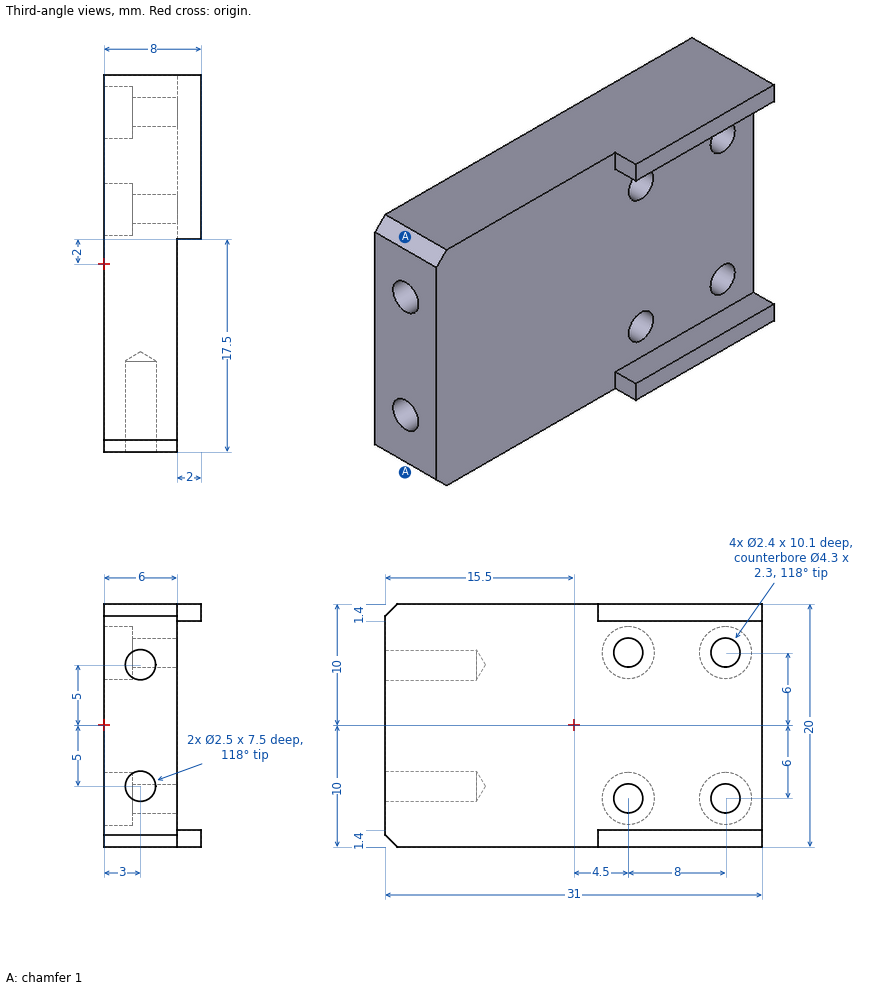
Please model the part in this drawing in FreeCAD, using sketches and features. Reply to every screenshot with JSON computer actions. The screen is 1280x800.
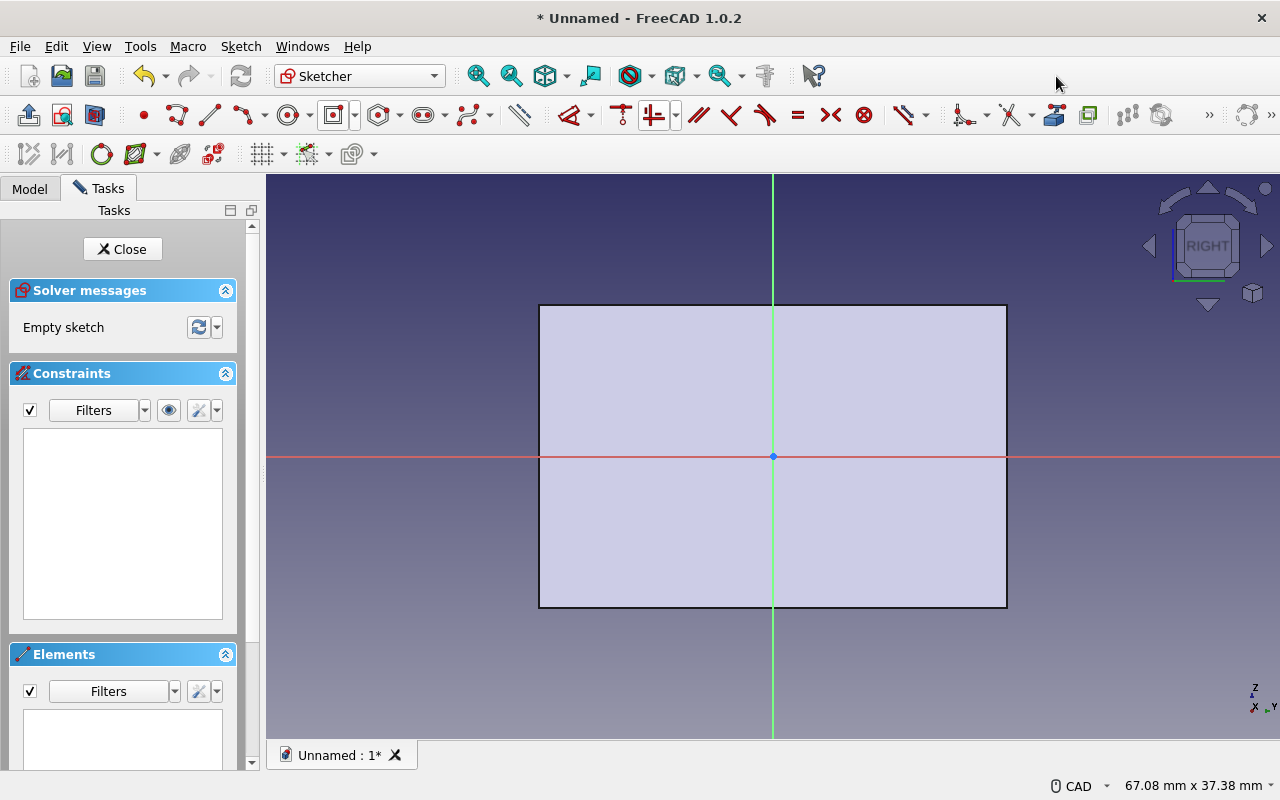
{"action": "key", "text": "g r"}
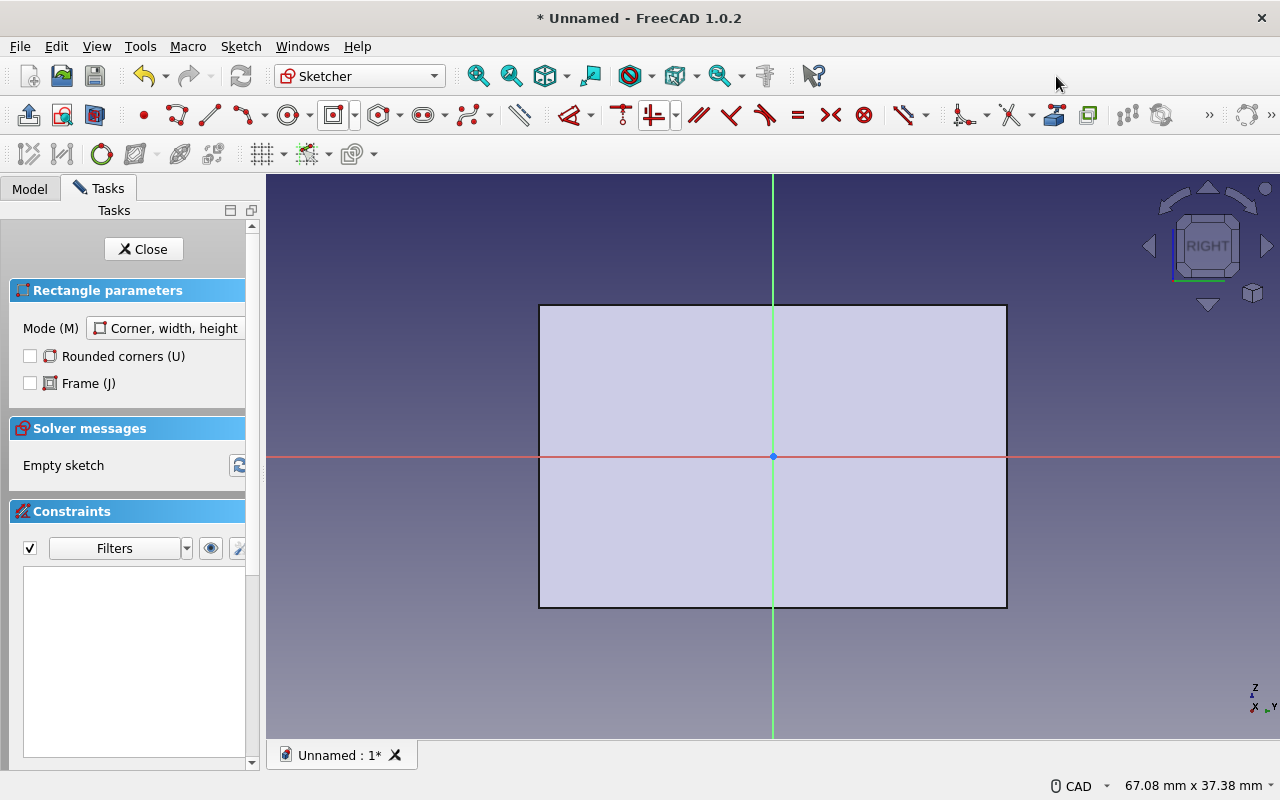
{"action": "left_click", "coordinate": [539, 305]}
{"action": "left_click", "coordinate": [1007, 326]}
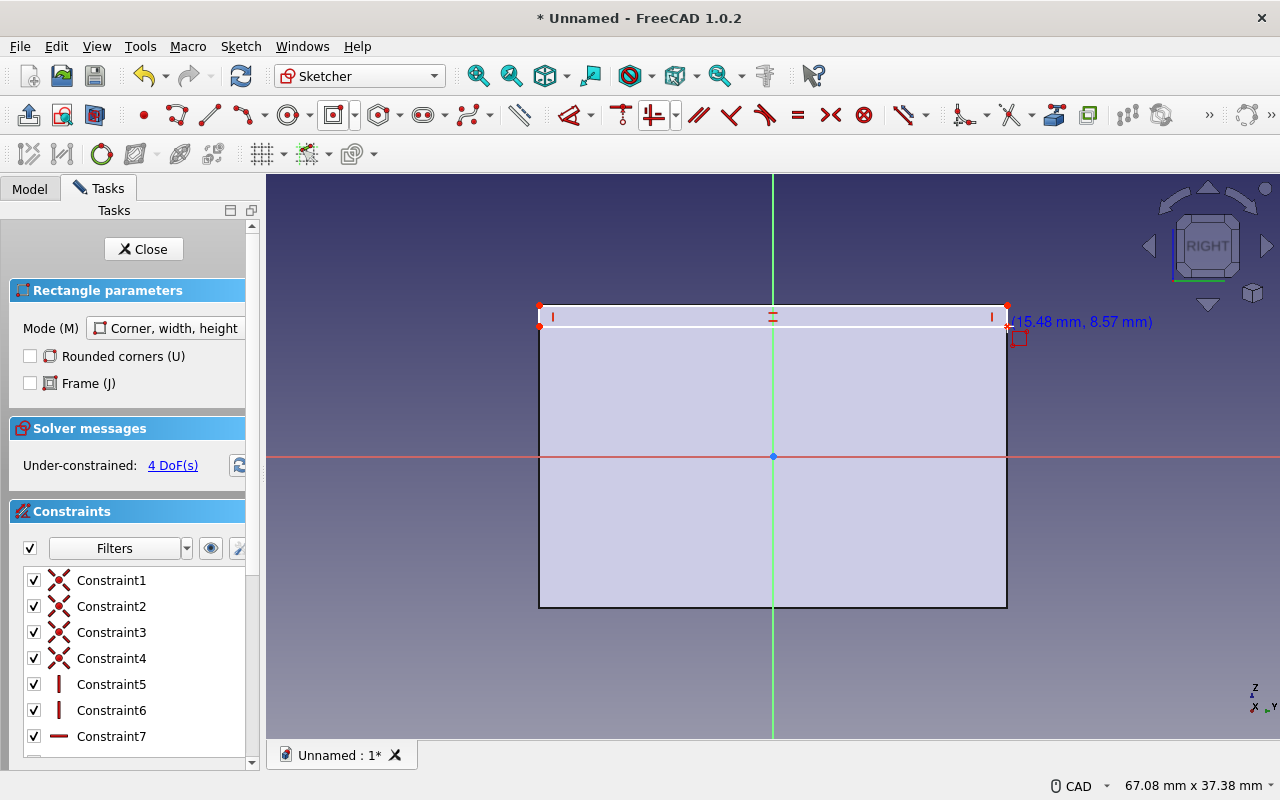
{"action": "left_click", "coordinate": [539, 587]}
{"action": "left_click", "coordinate": [1007, 608]}
{"action": "key", "text": "Escape"}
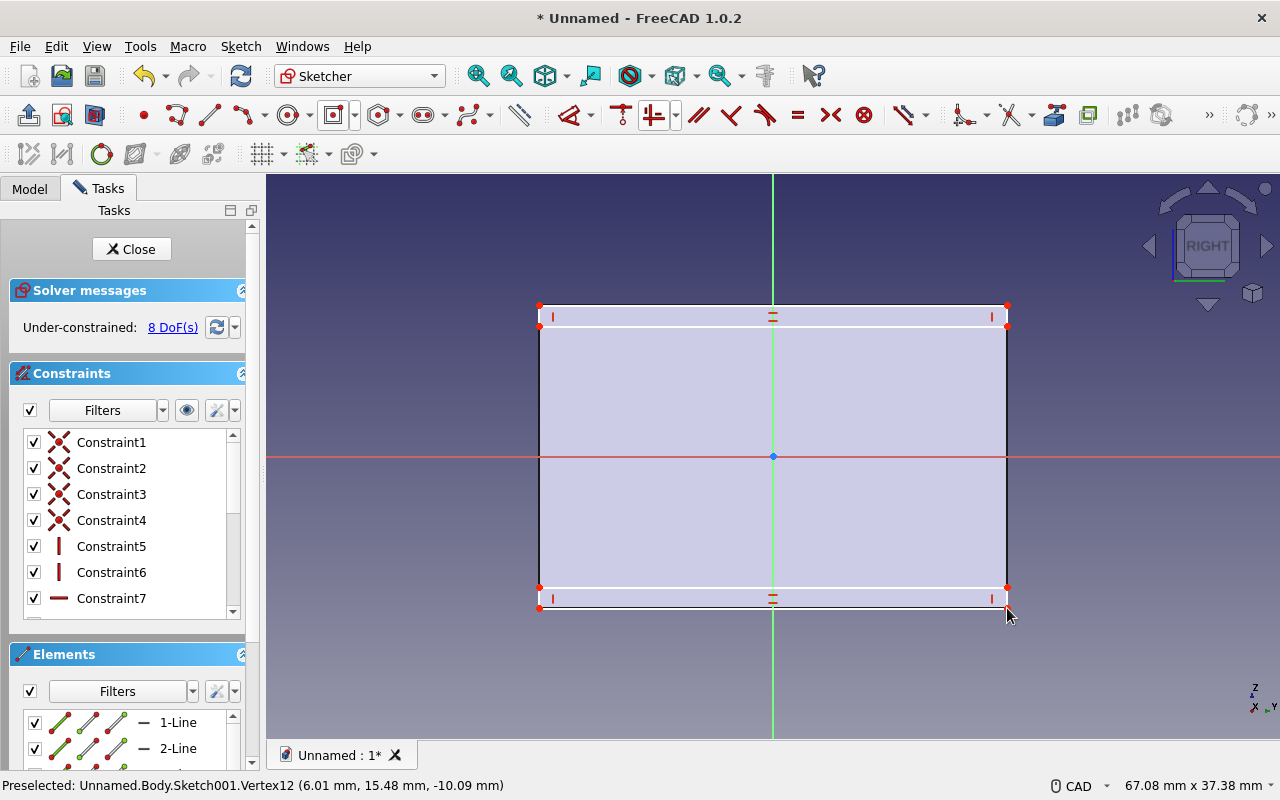
{"action": "left_click", "coordinate": [568, 116]}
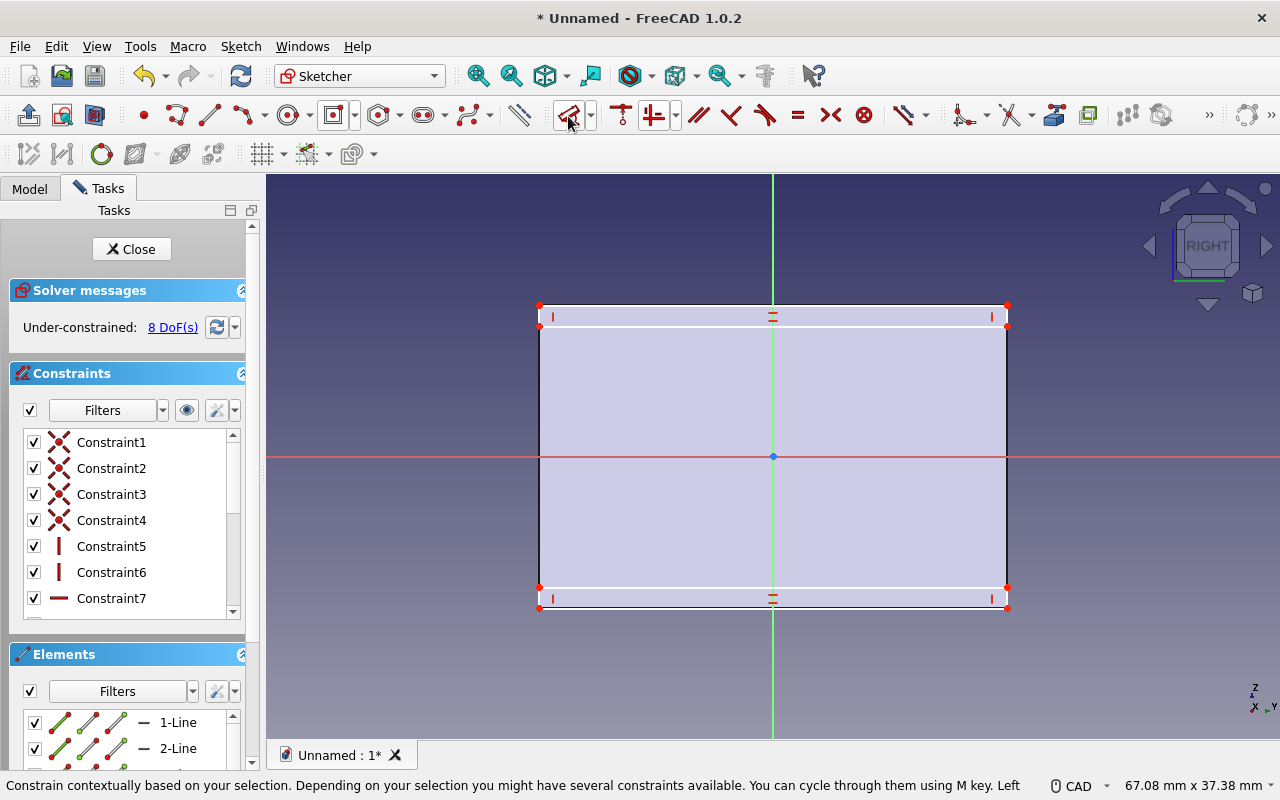
{"action": "left_click", "coordinate": [679, 327]}
{"action": "left_click", "coordinate": [665, 361]}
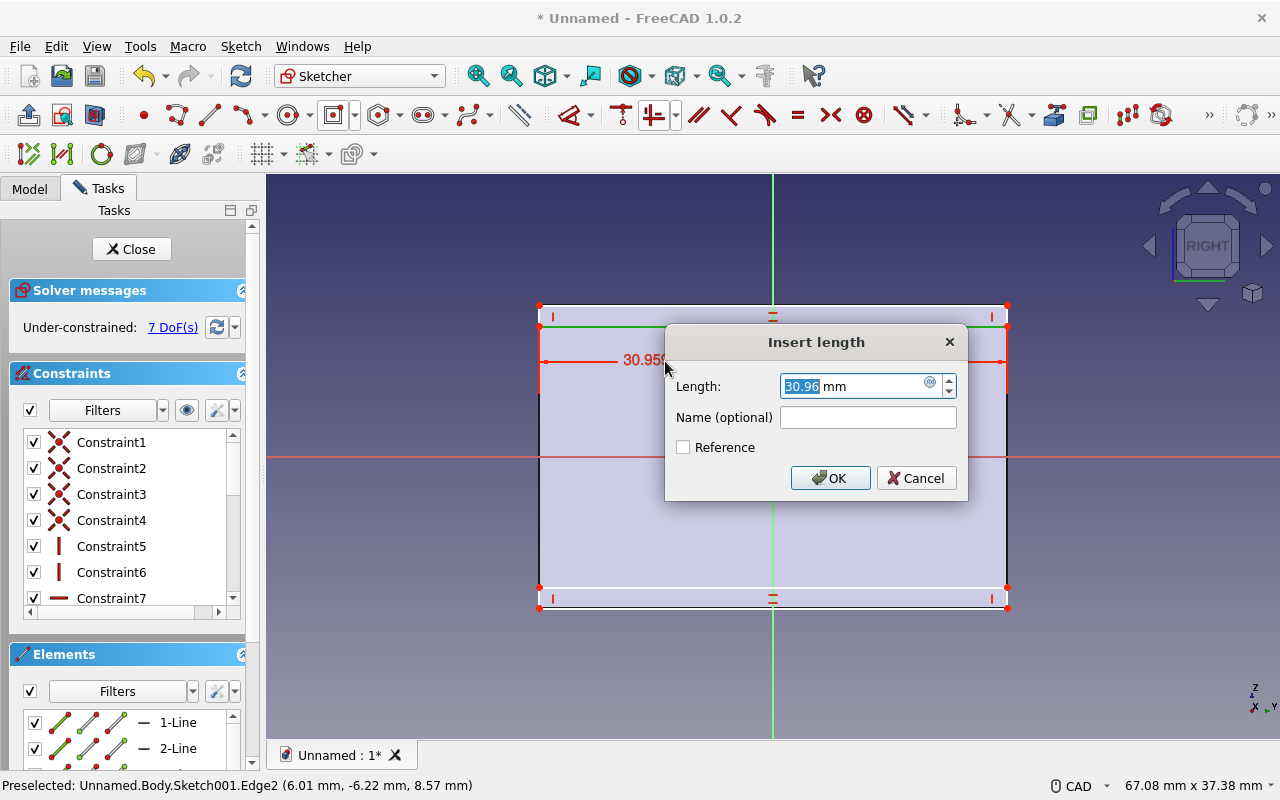
{"action": "type", "text": "31"}
{"action": "key", "text": "Return"}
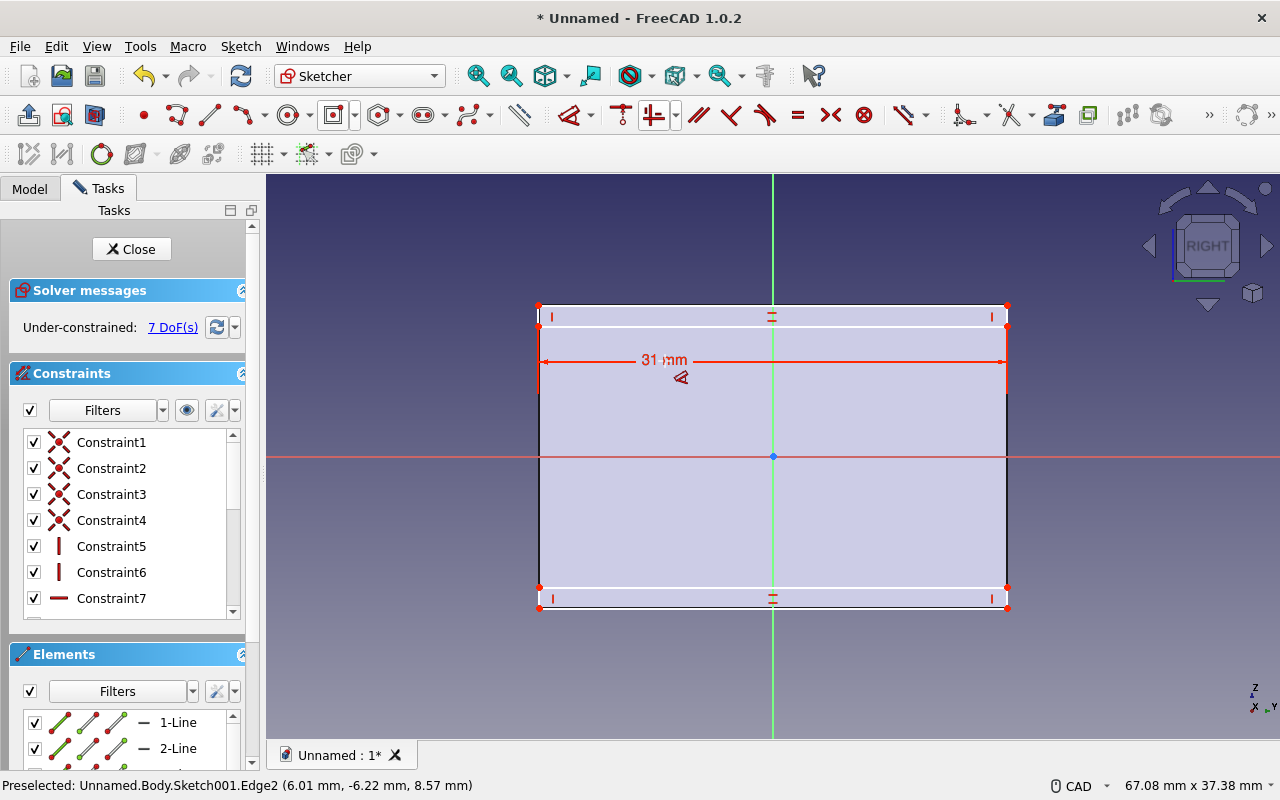
{"action": "left_click", "coordinate": [679, 609]}
{"action": "left_click", "coordinate": [665, 643]}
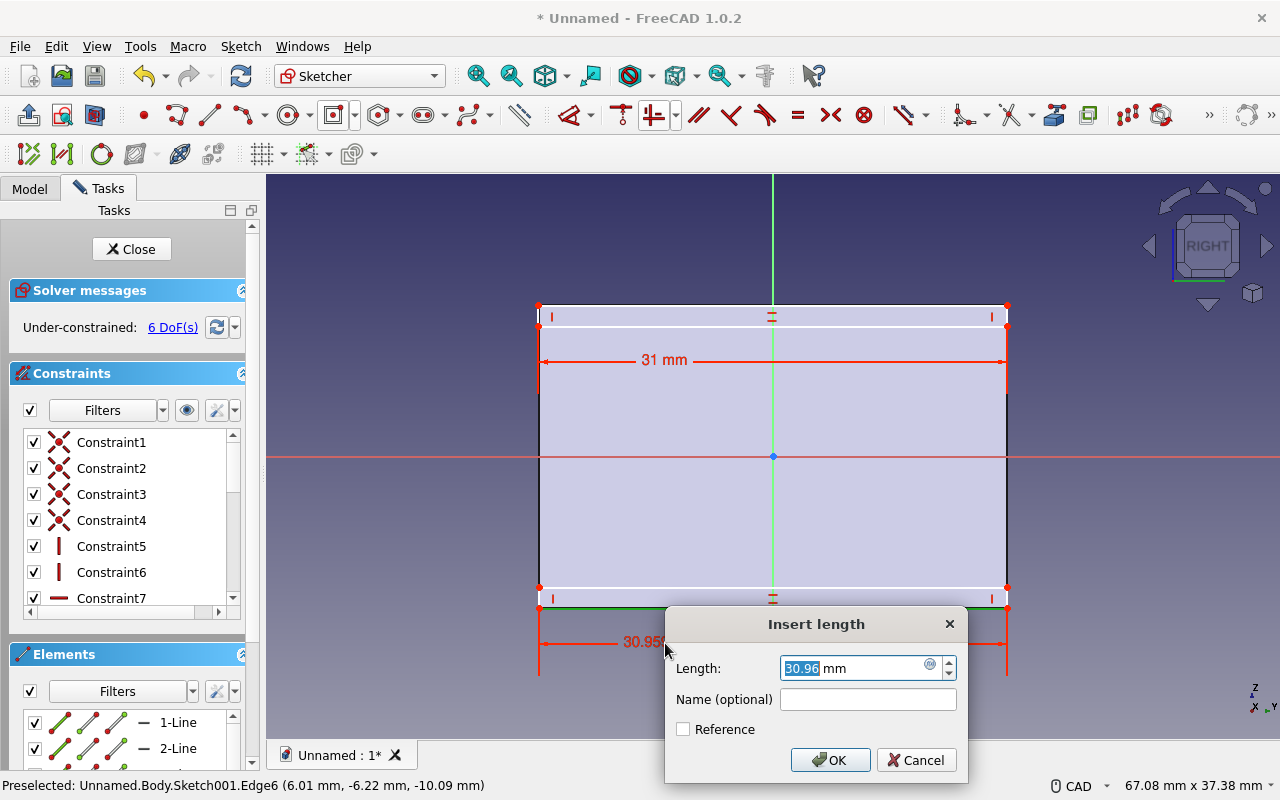
{"action": "type", "text": "31"}
{"action": "key", "text": "Return"}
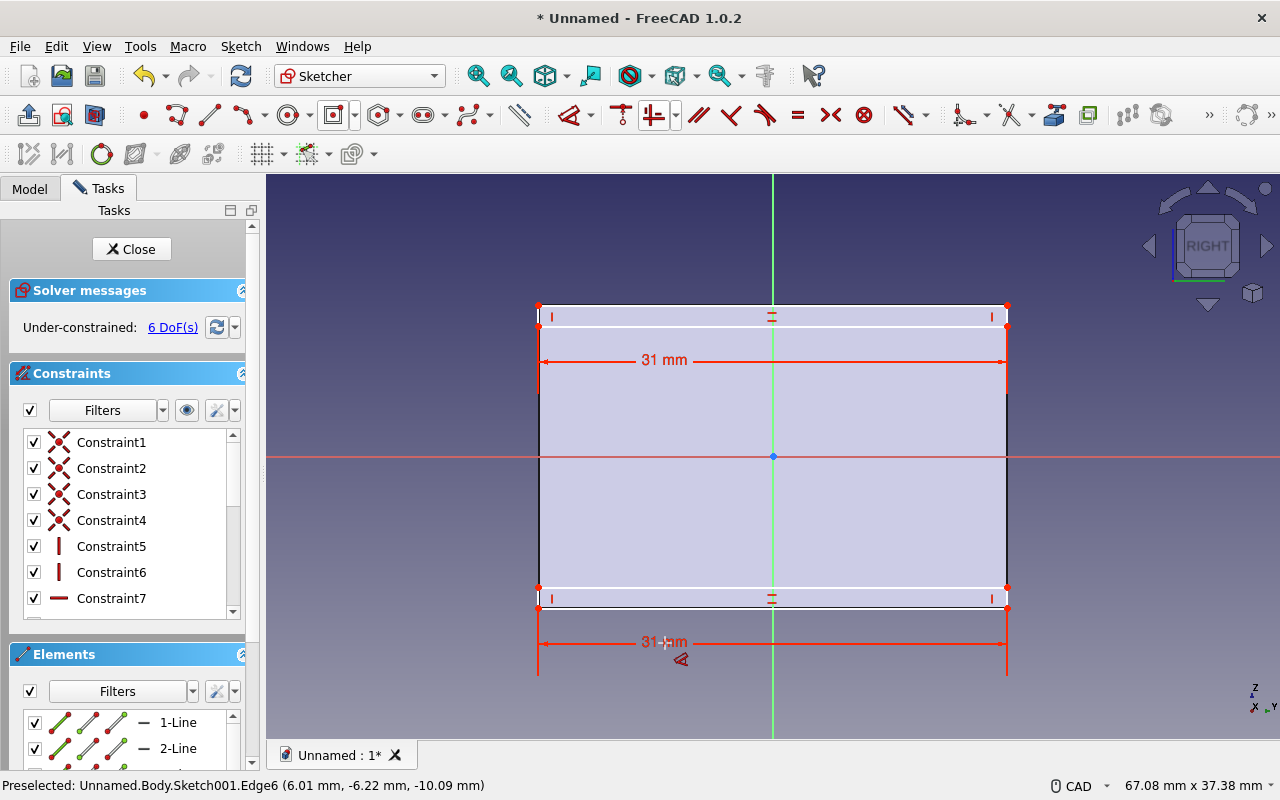
{"action": "scroll", "coordinate": [538, 317], "scroll_direction": "up", "scroll_amount": 4}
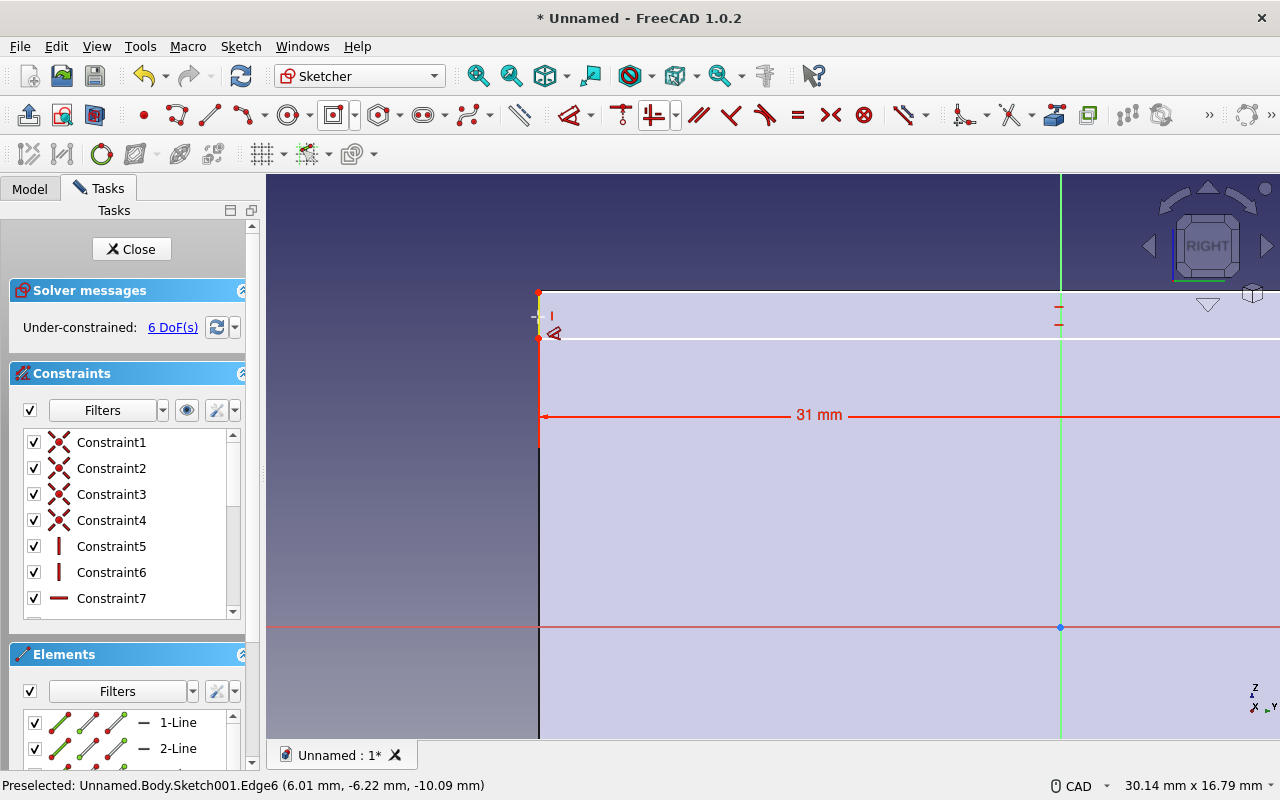
{"action": "left_click", "coordinate": [539, 316]}
{"action": "left_click", "coordinate": [505, 316]}